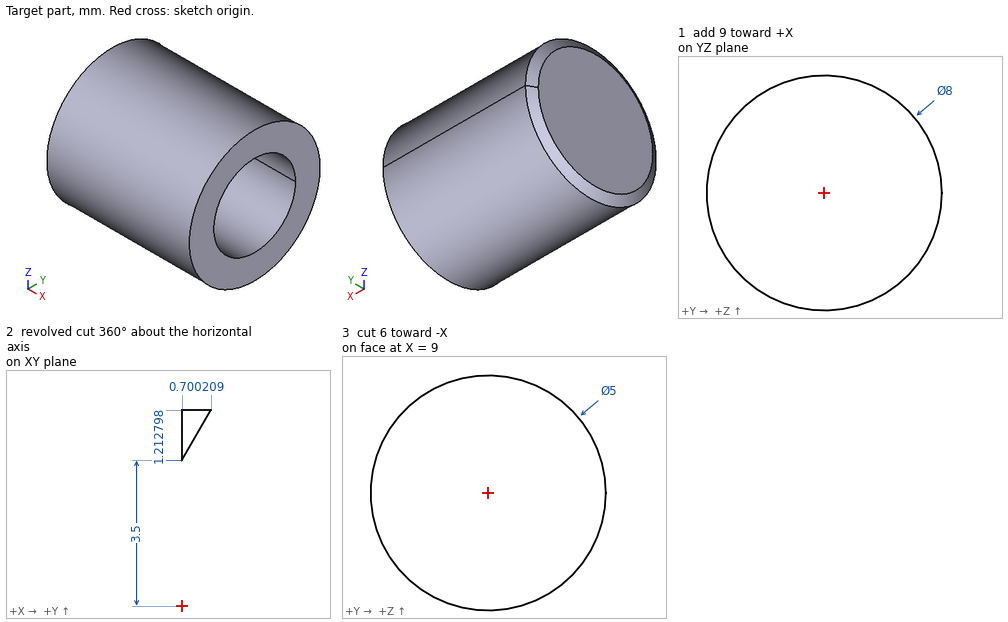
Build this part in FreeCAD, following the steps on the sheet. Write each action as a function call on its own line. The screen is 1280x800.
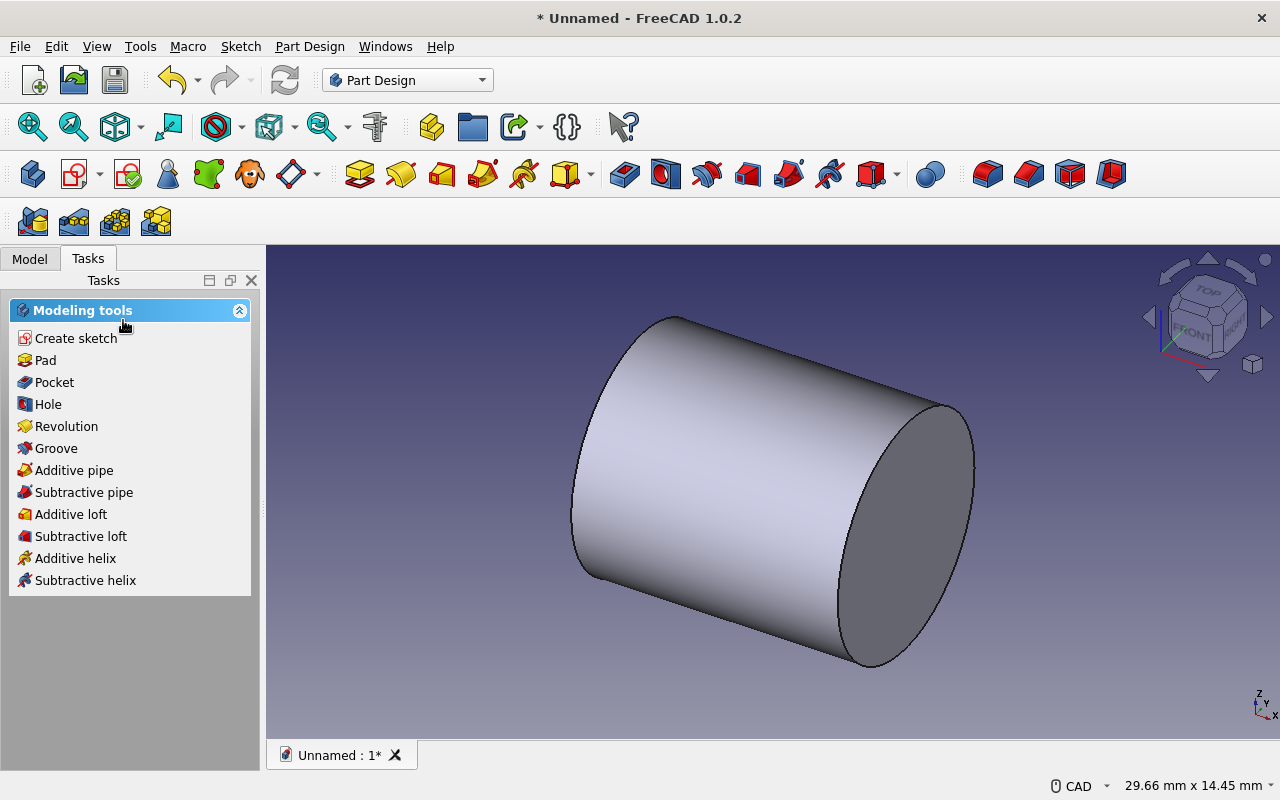
click(707, 174)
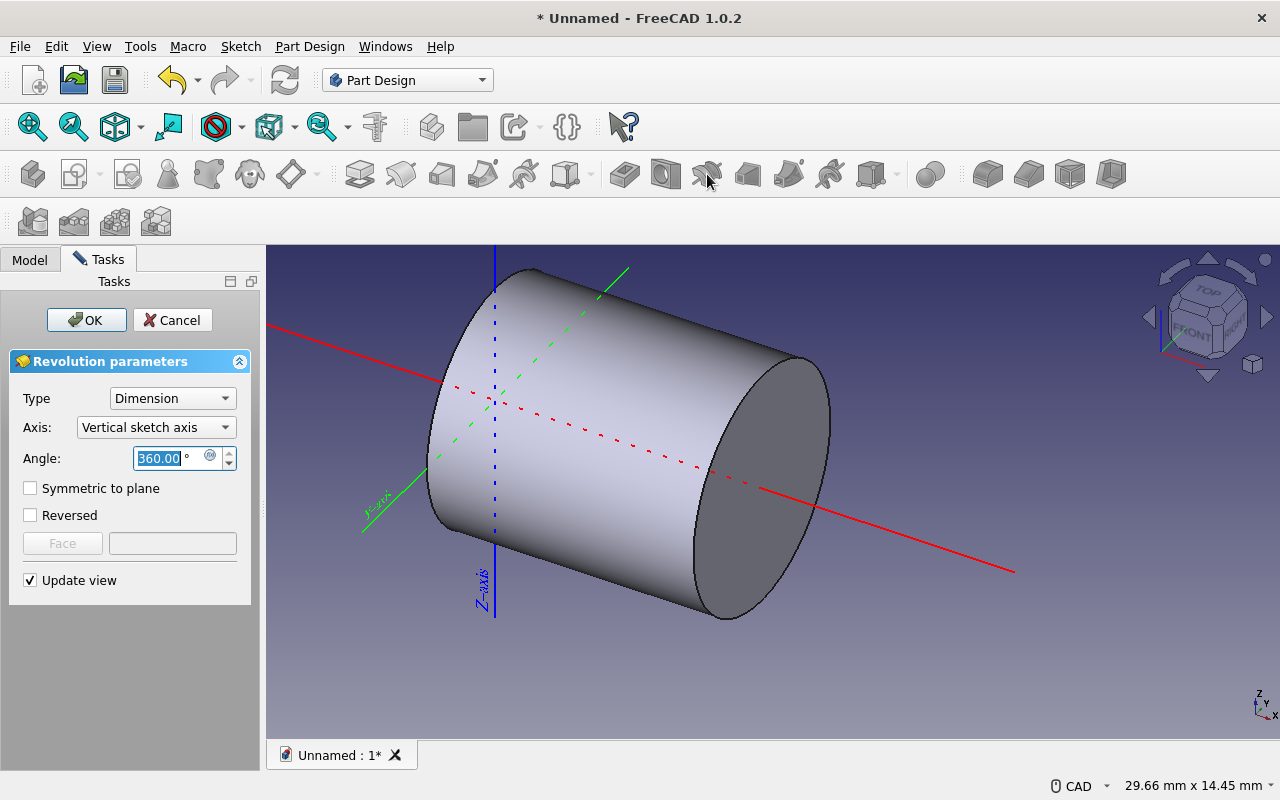
click(157, 428)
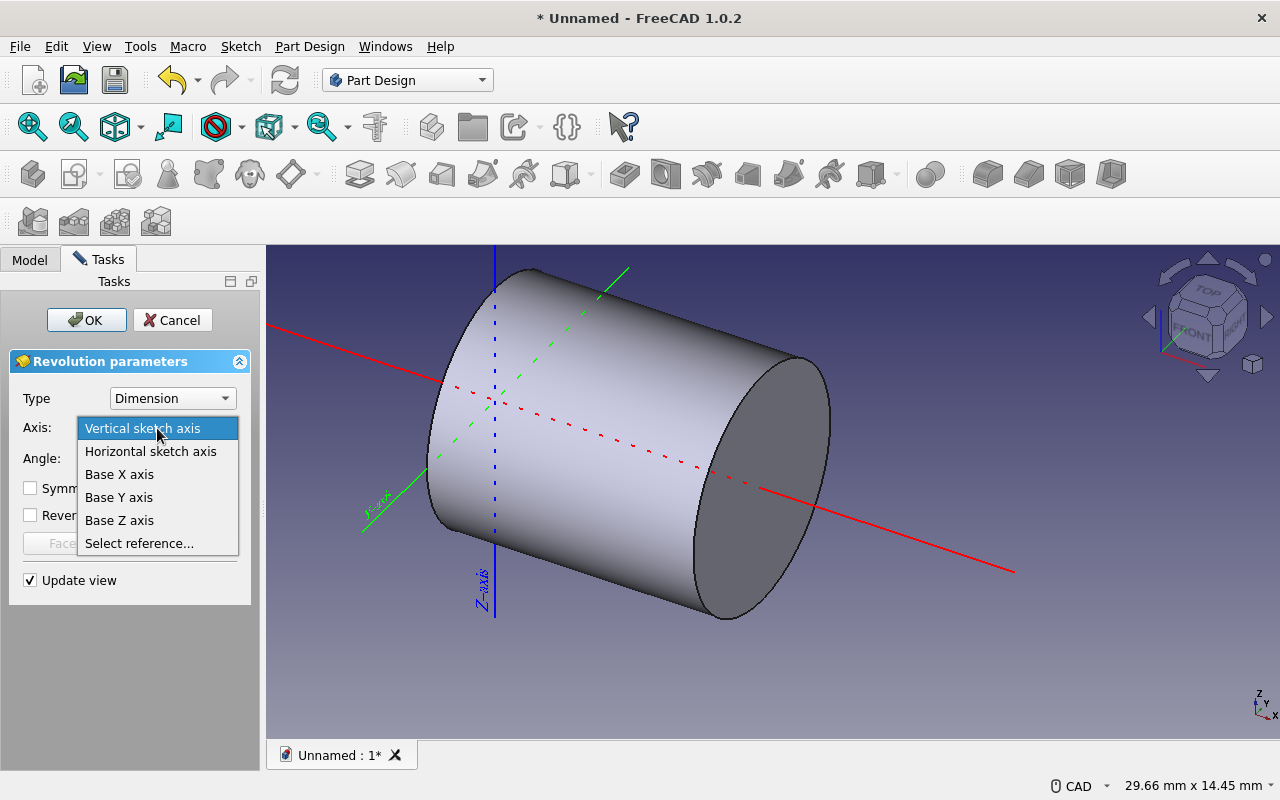
click(156, 452)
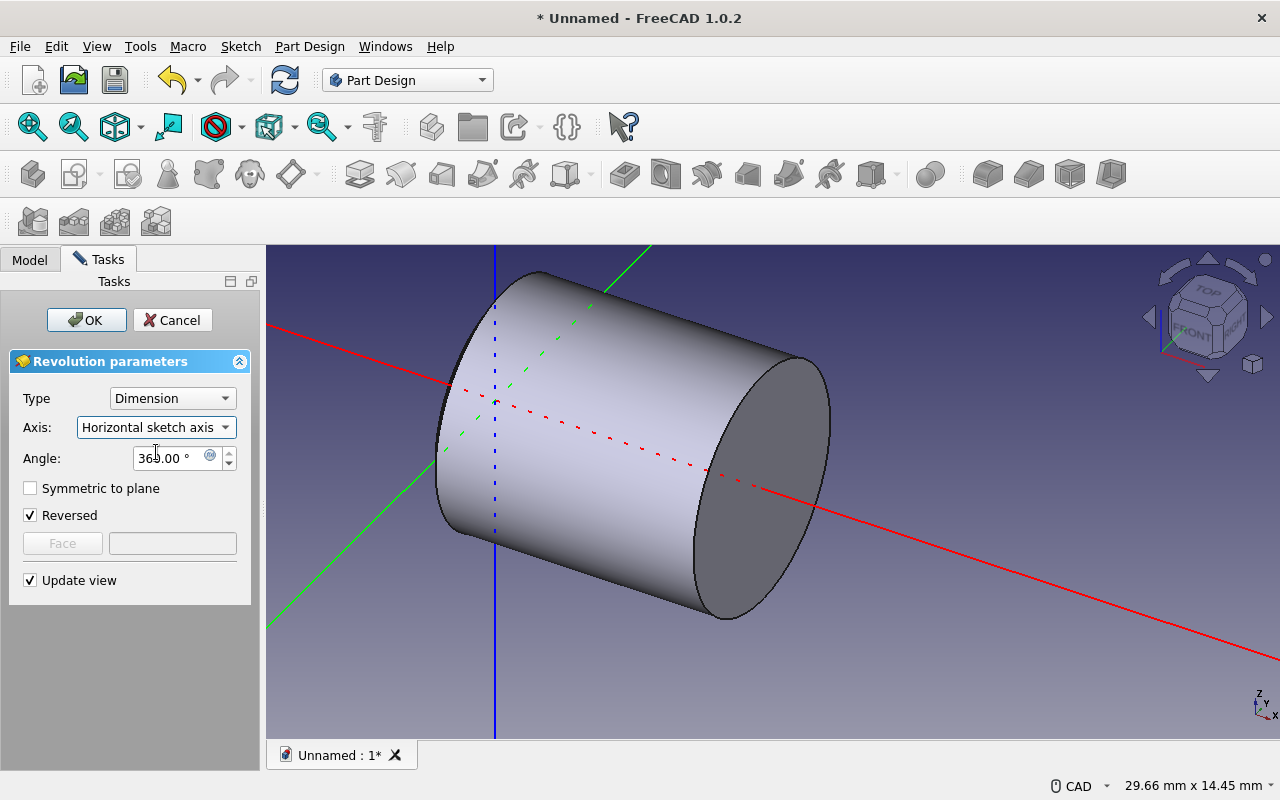
click(87, 320)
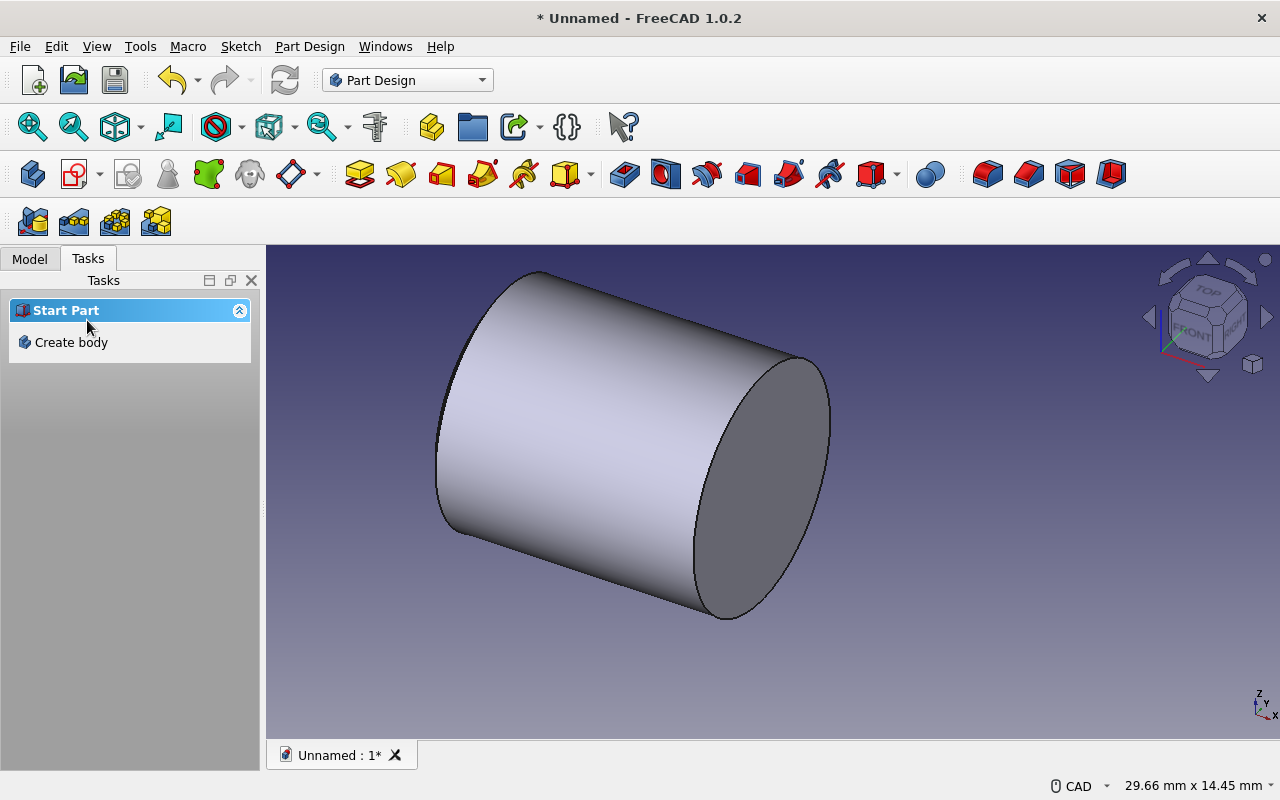
click(33, 128)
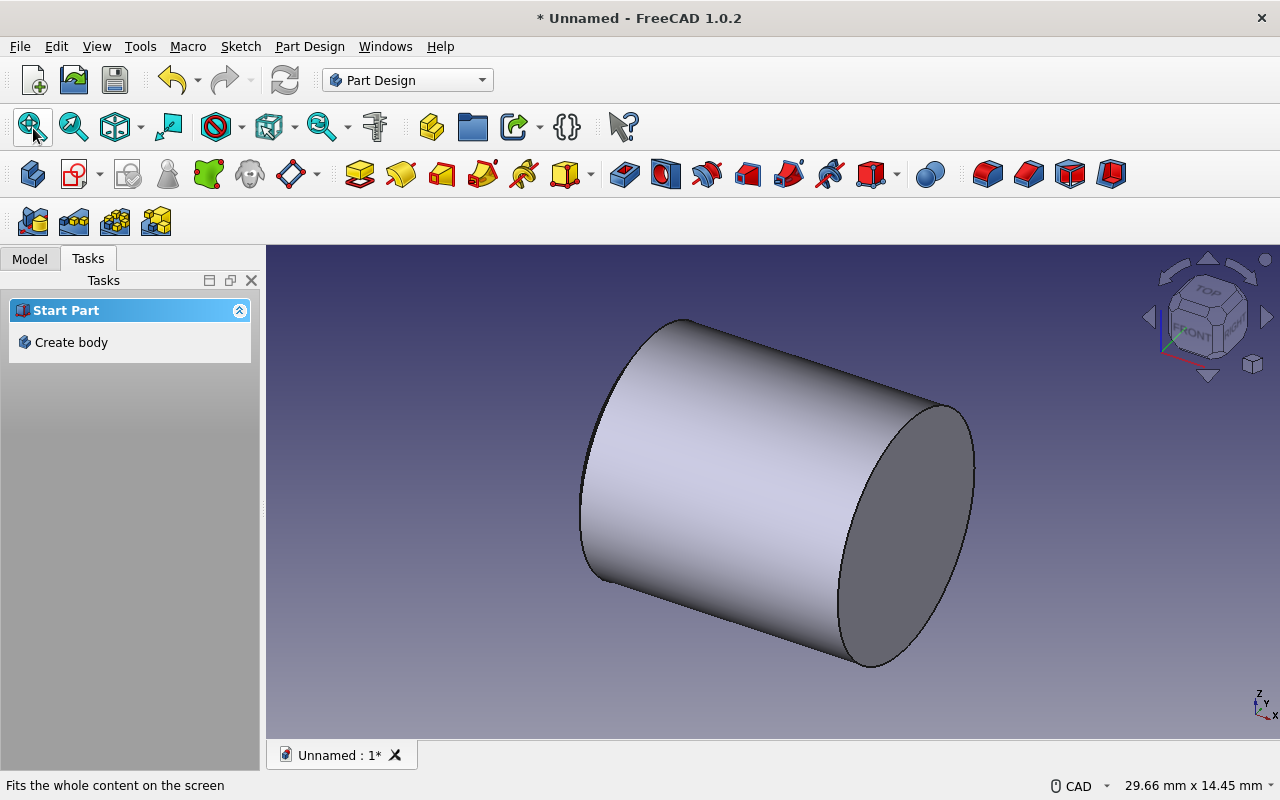
click(906, 535)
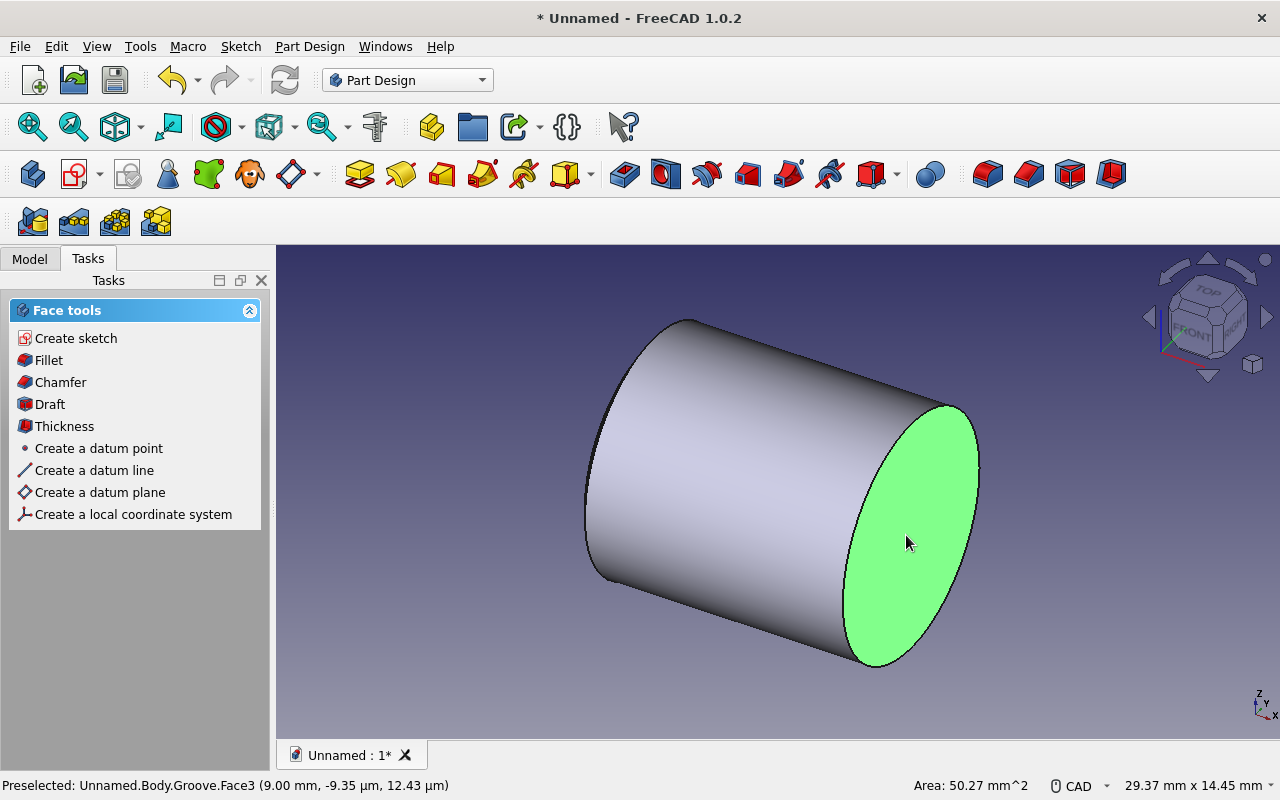
click(74, 174)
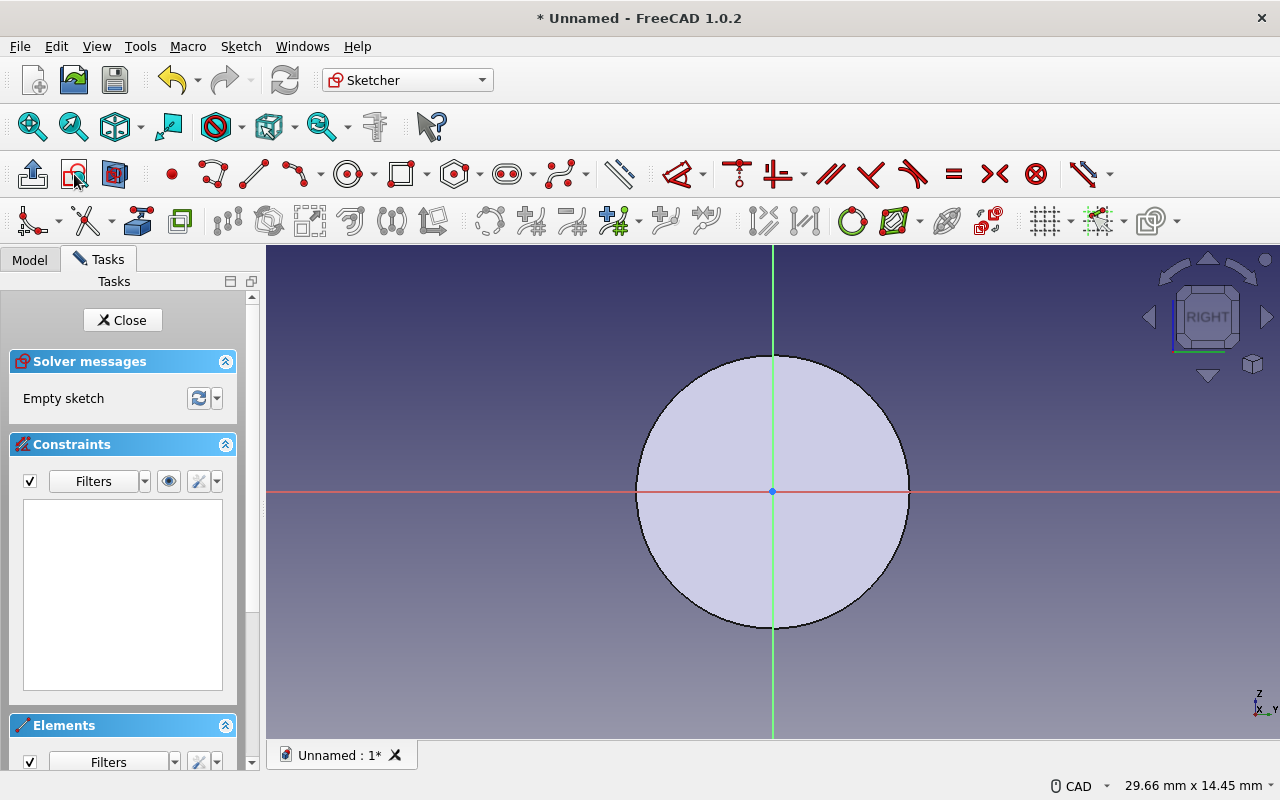
scroll(856, 492, up, 3)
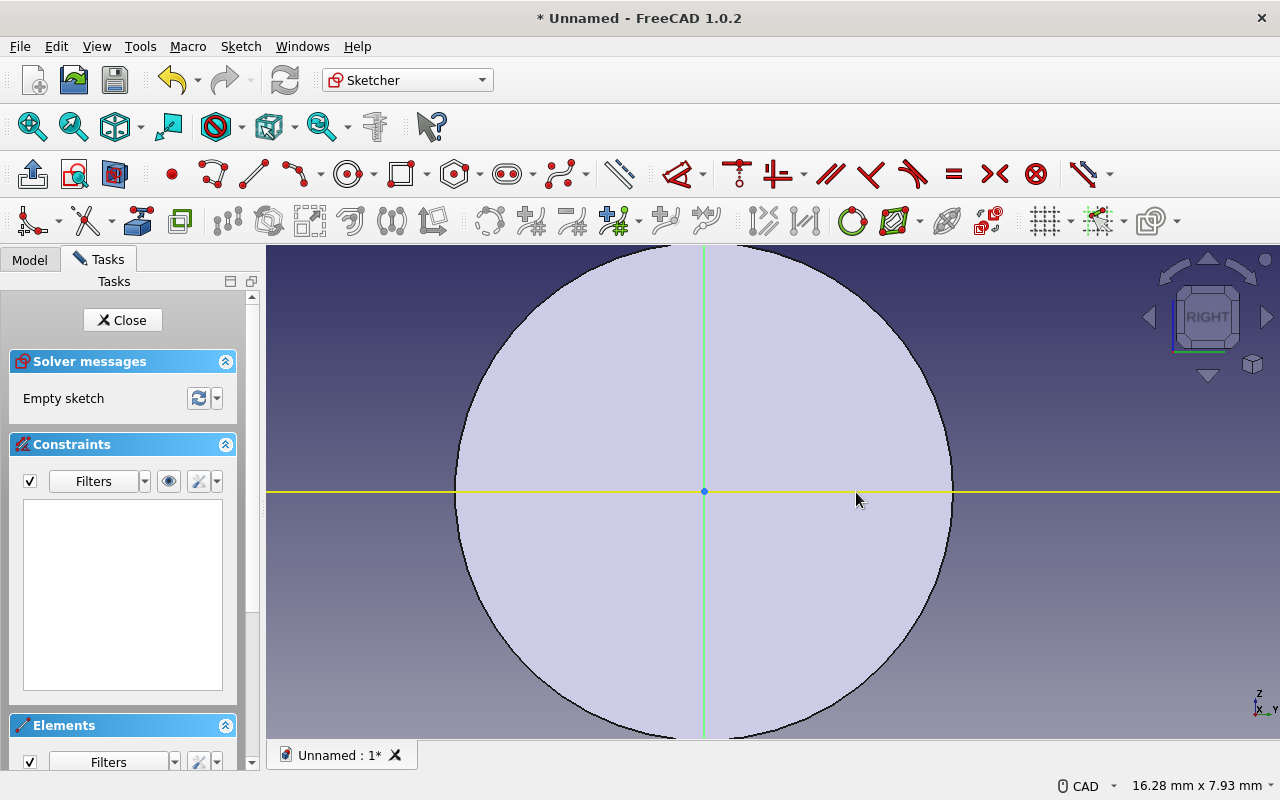
click(348, 174)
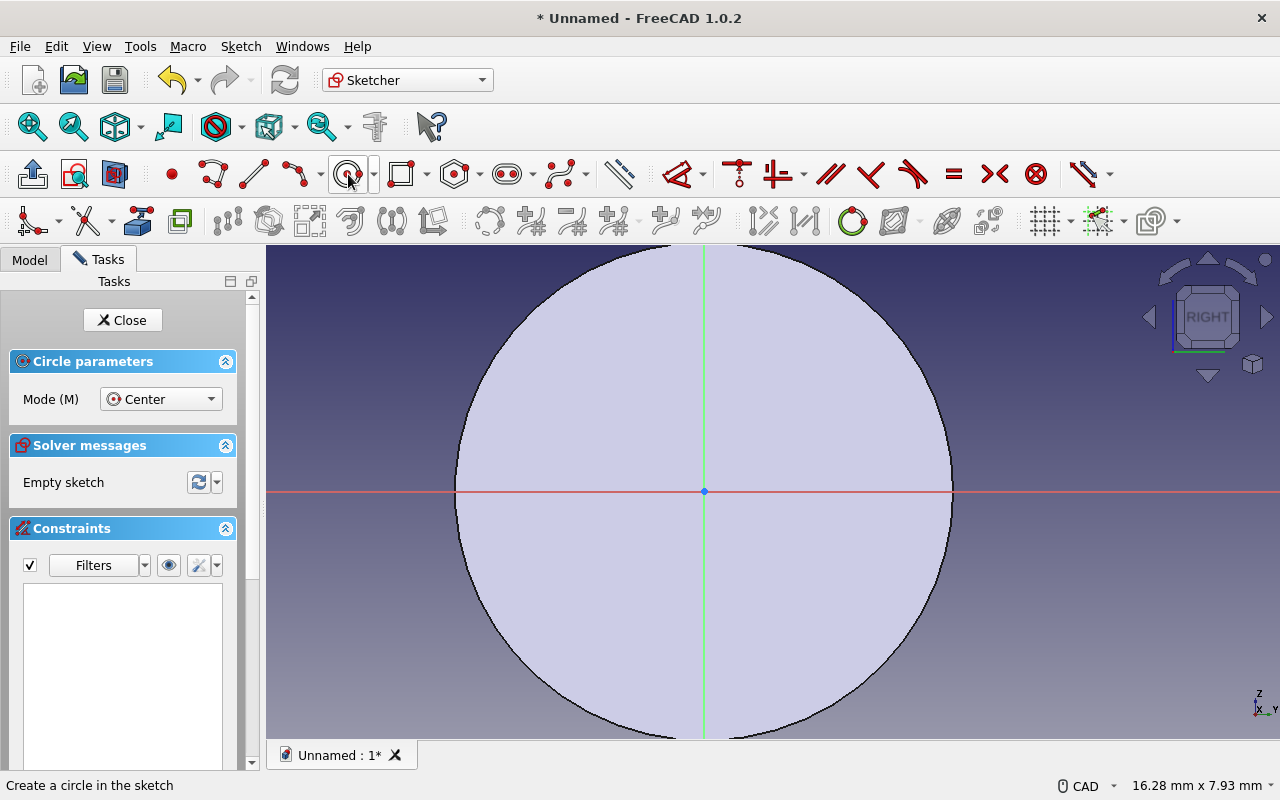
click(704, 492)
click(814, 381)
key(Escape)